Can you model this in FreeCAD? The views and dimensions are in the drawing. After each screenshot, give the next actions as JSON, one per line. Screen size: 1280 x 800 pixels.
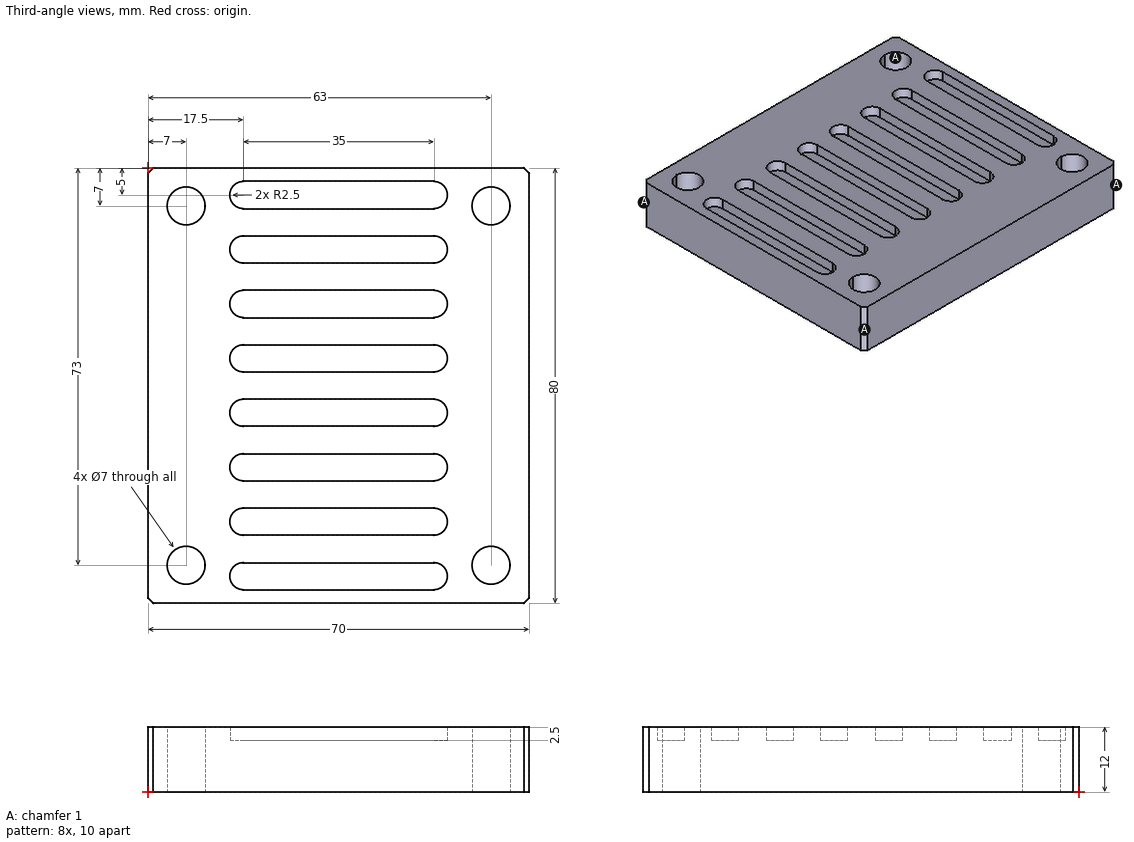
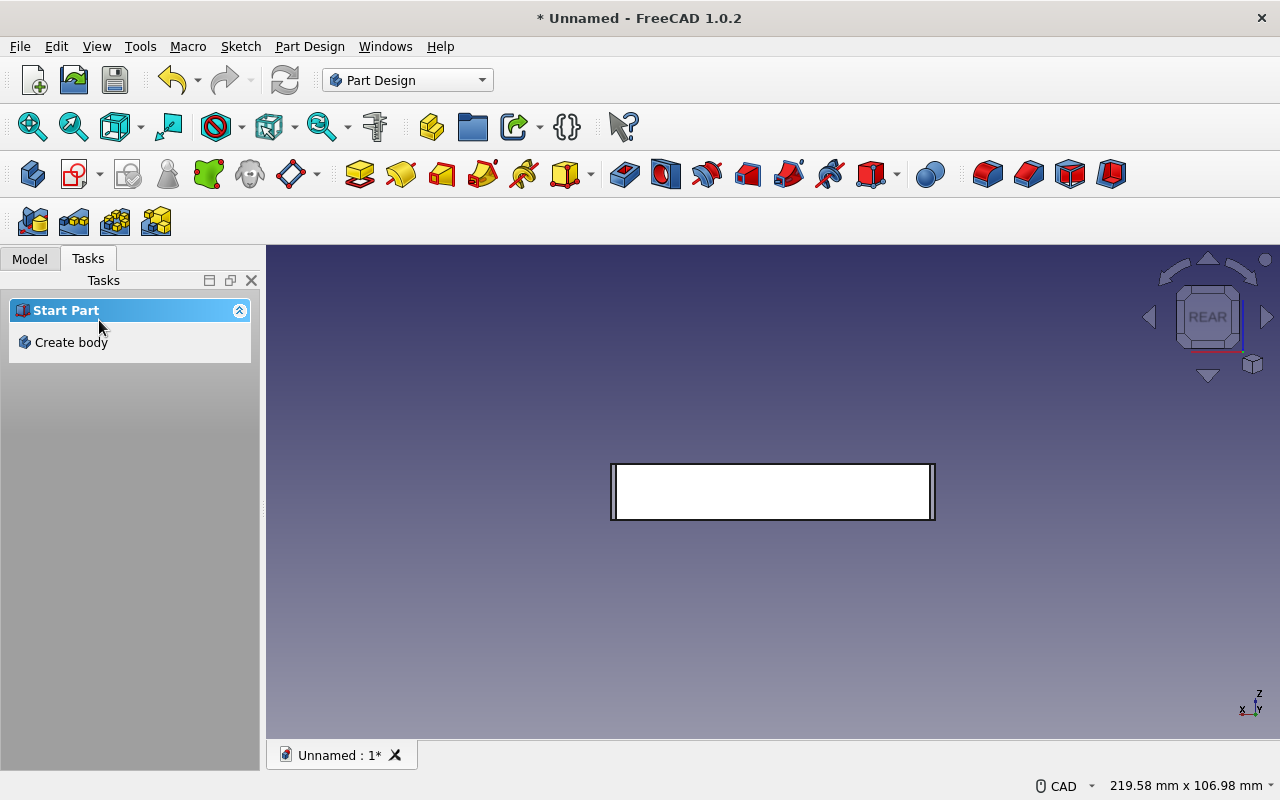
{"action": "key", "text": "0"}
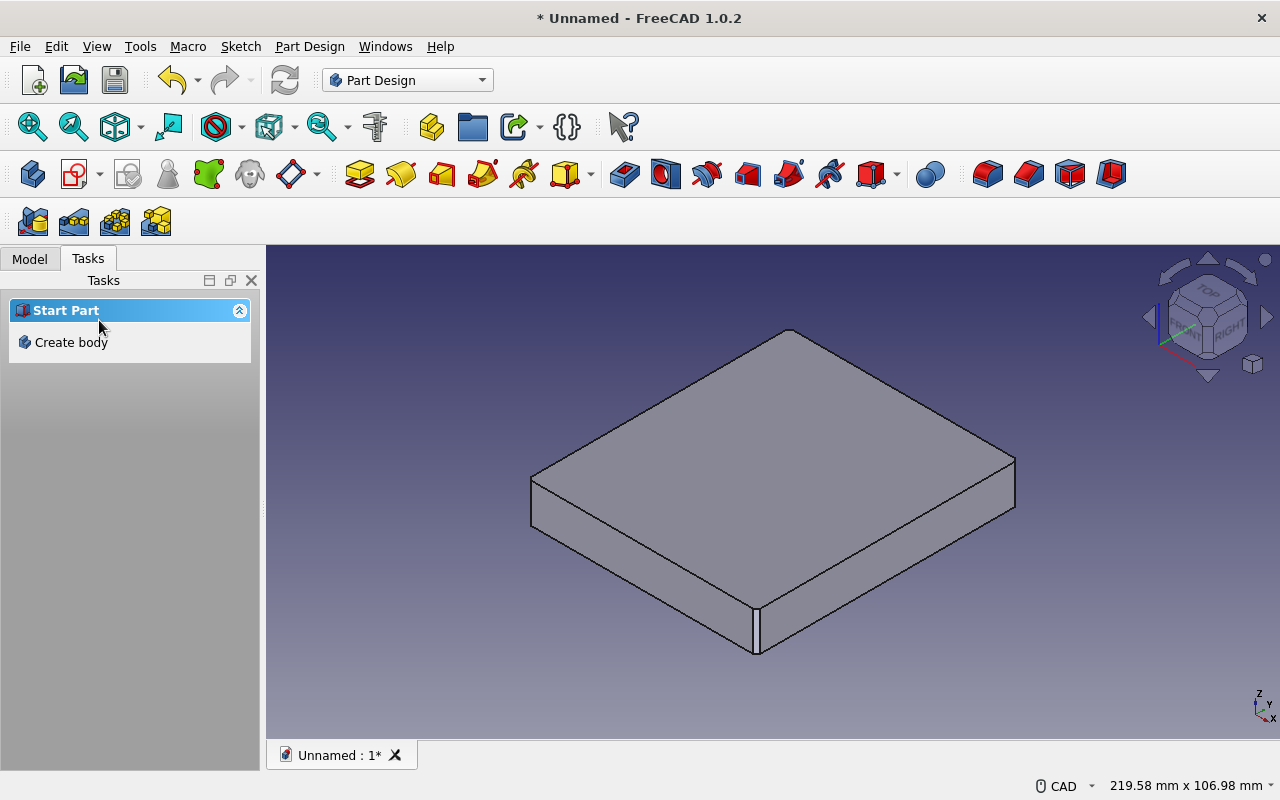
{"action": "left_click", "coordinate": [773, 468]}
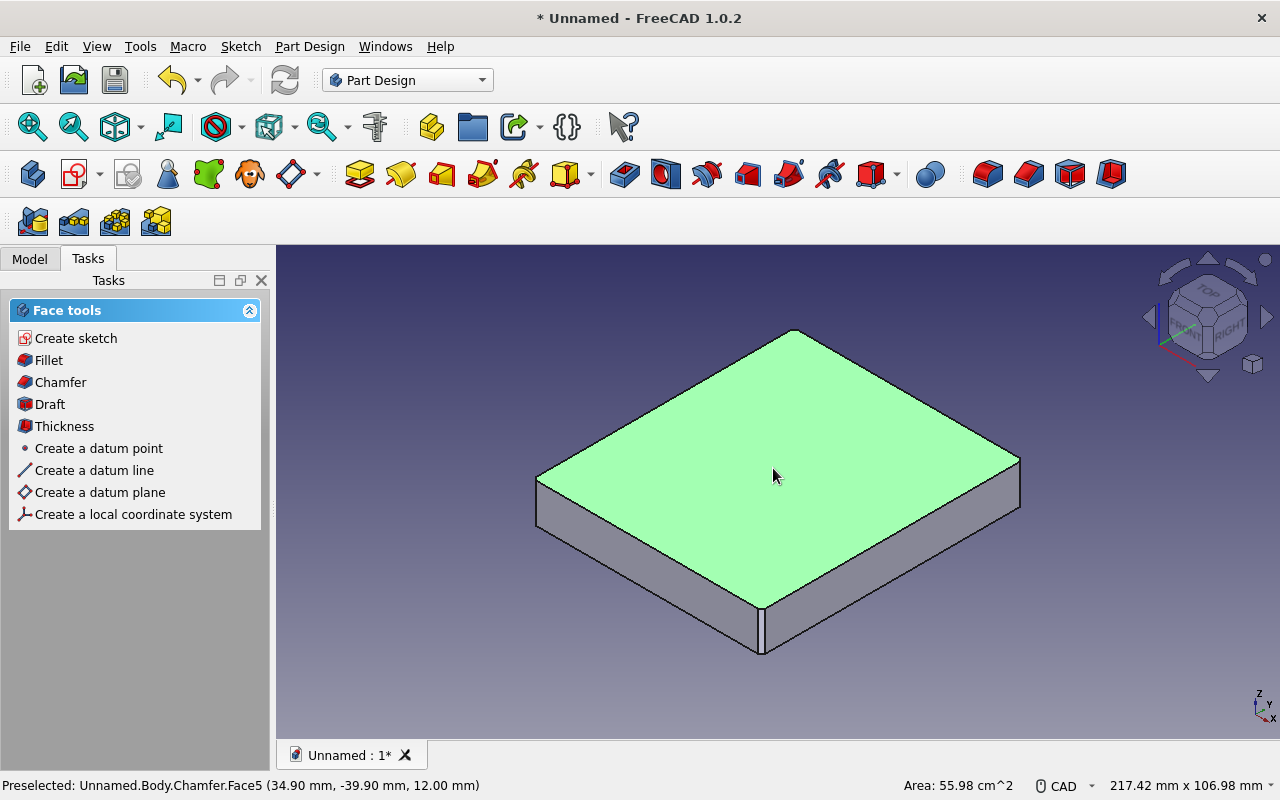
{"action": "left_click", "coordinate": [74, 174]}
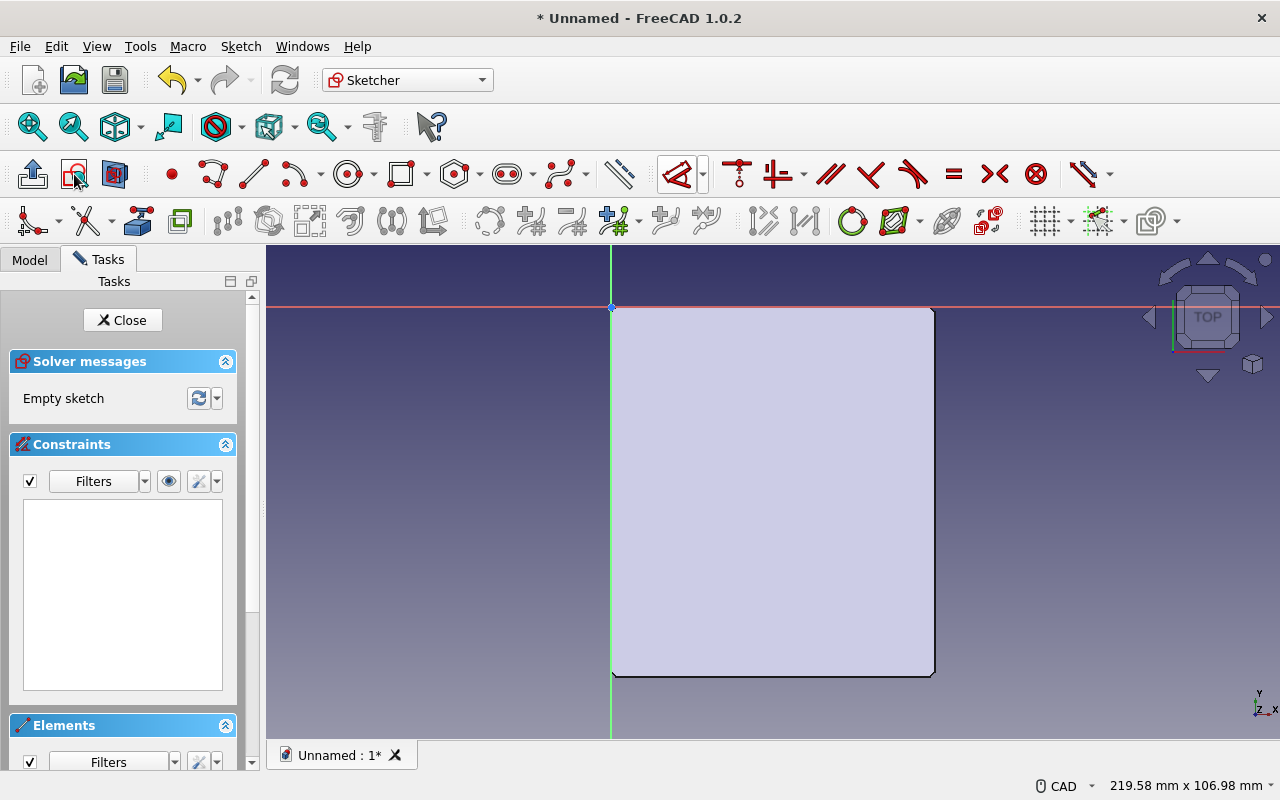
{"action": "scroll", "coordinate": [766, 273], "scroll_direction": "up", "scroll_amount": 4}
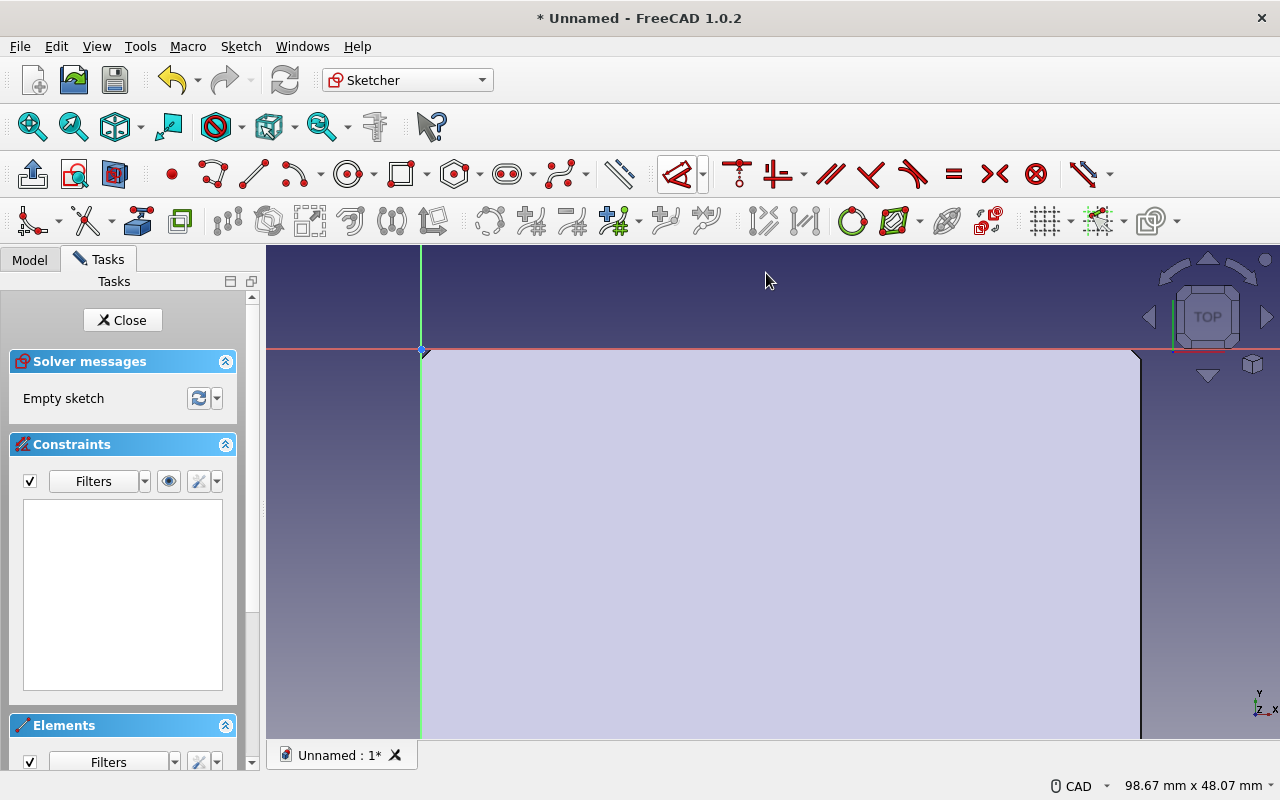
{"action": "key", "text": "g s"}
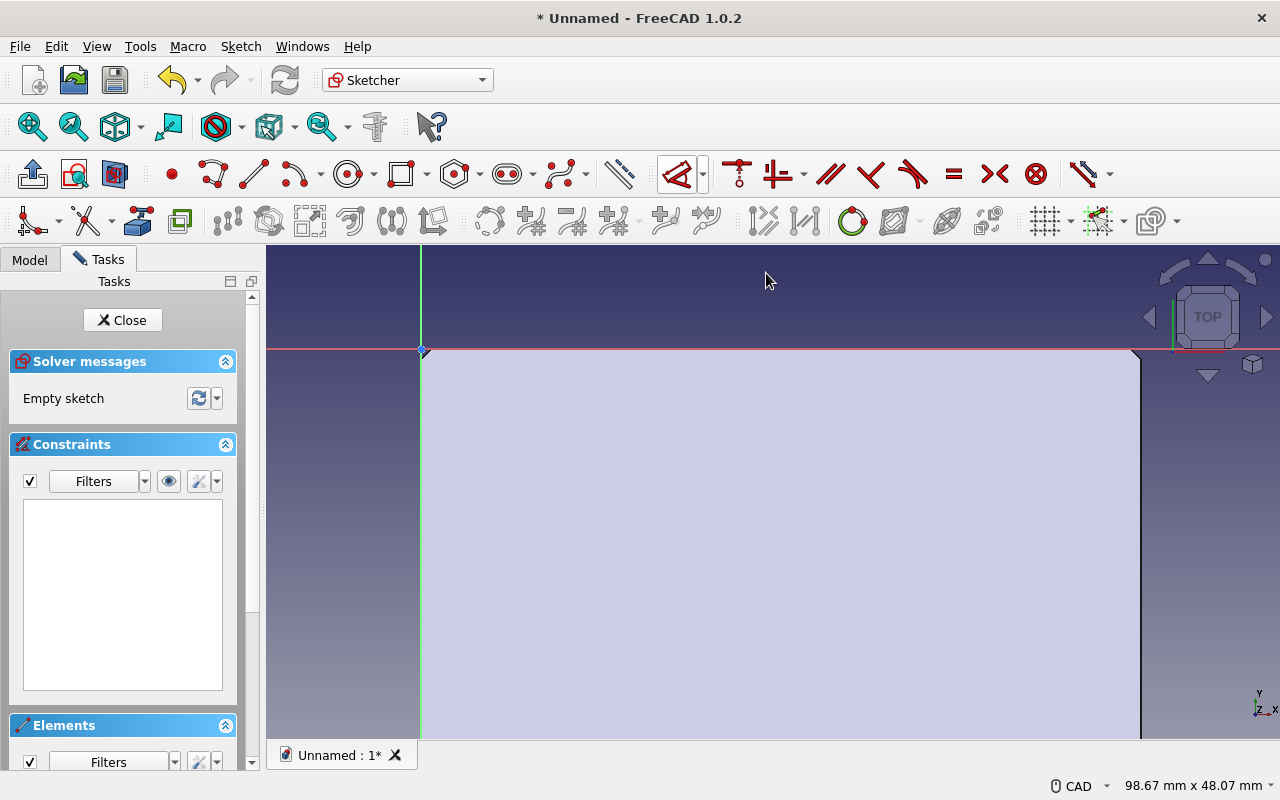
{"action": "left_click", "coordinate": [601, 401]}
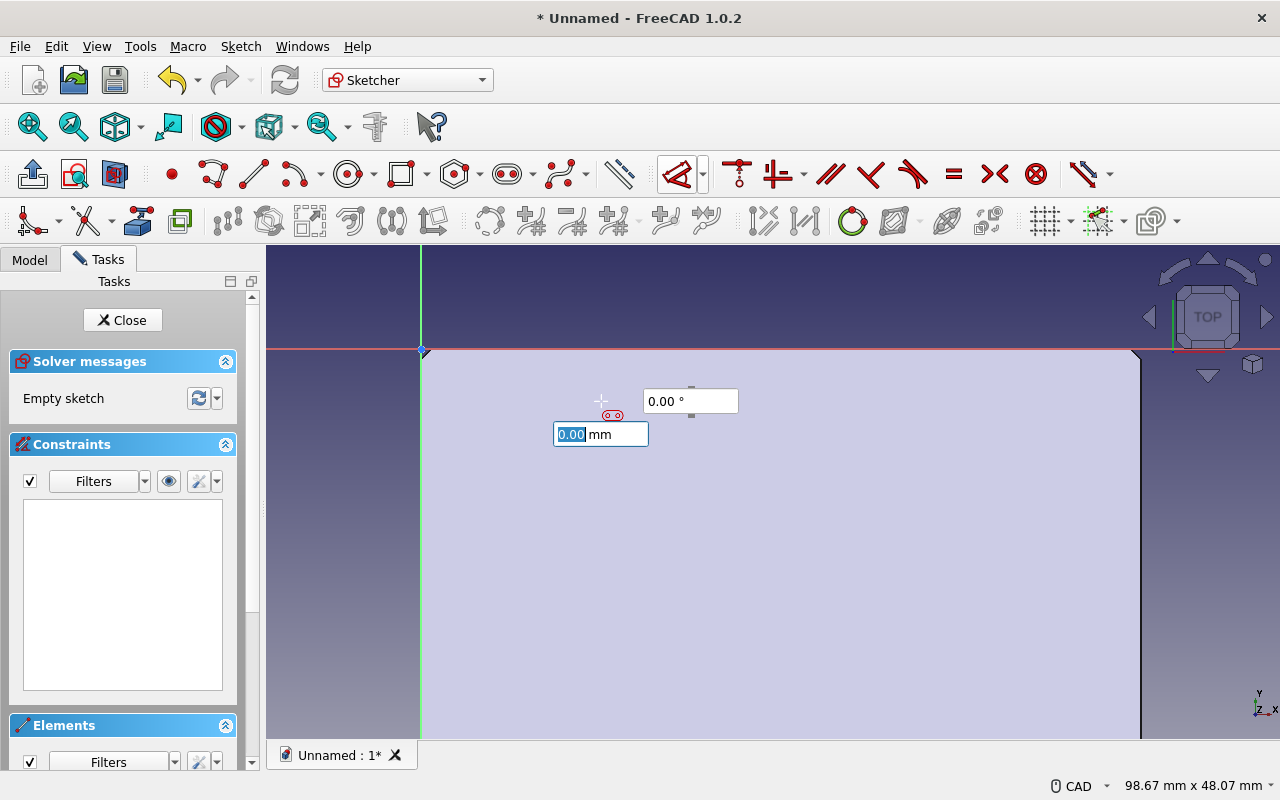
{"action": "left_click", "coordinate": [961, 401]}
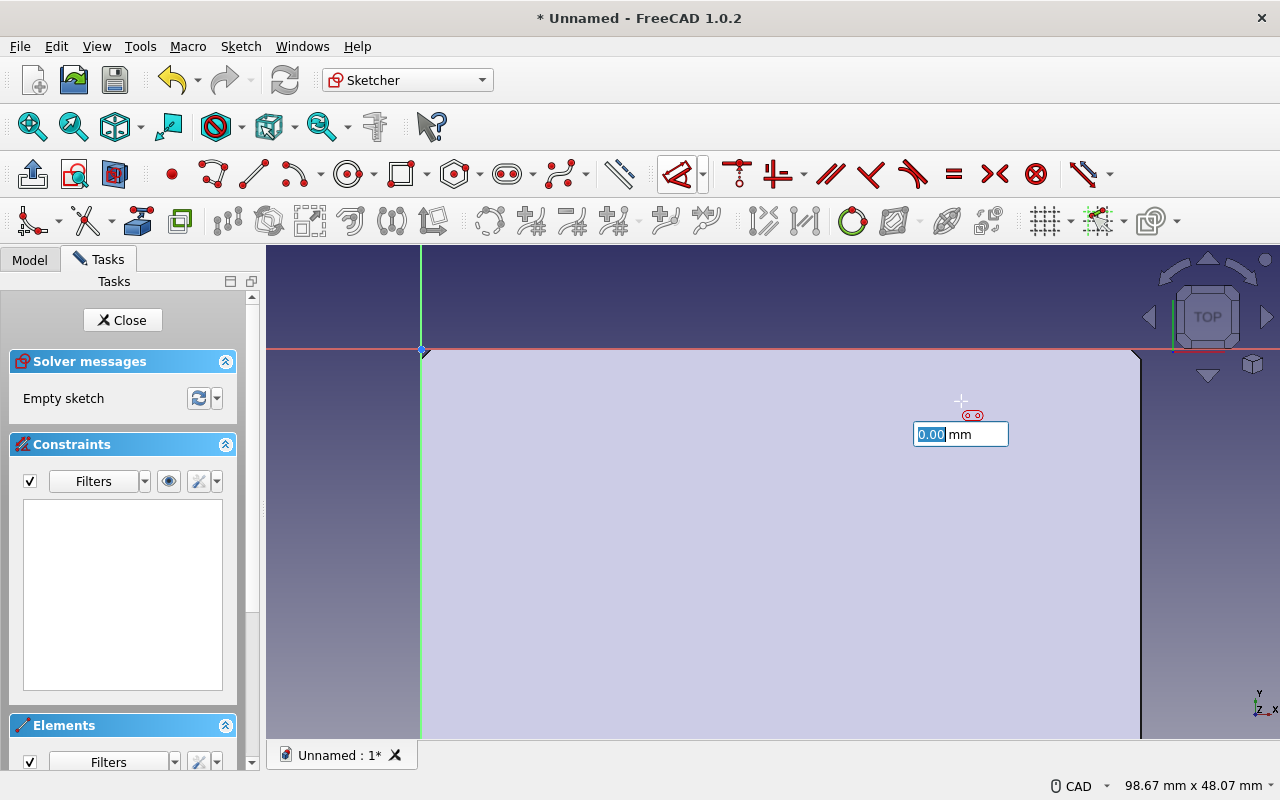
{"action": "left_click", "coordinate": [781, 375]}
{"action": "key", "text": "Escape"}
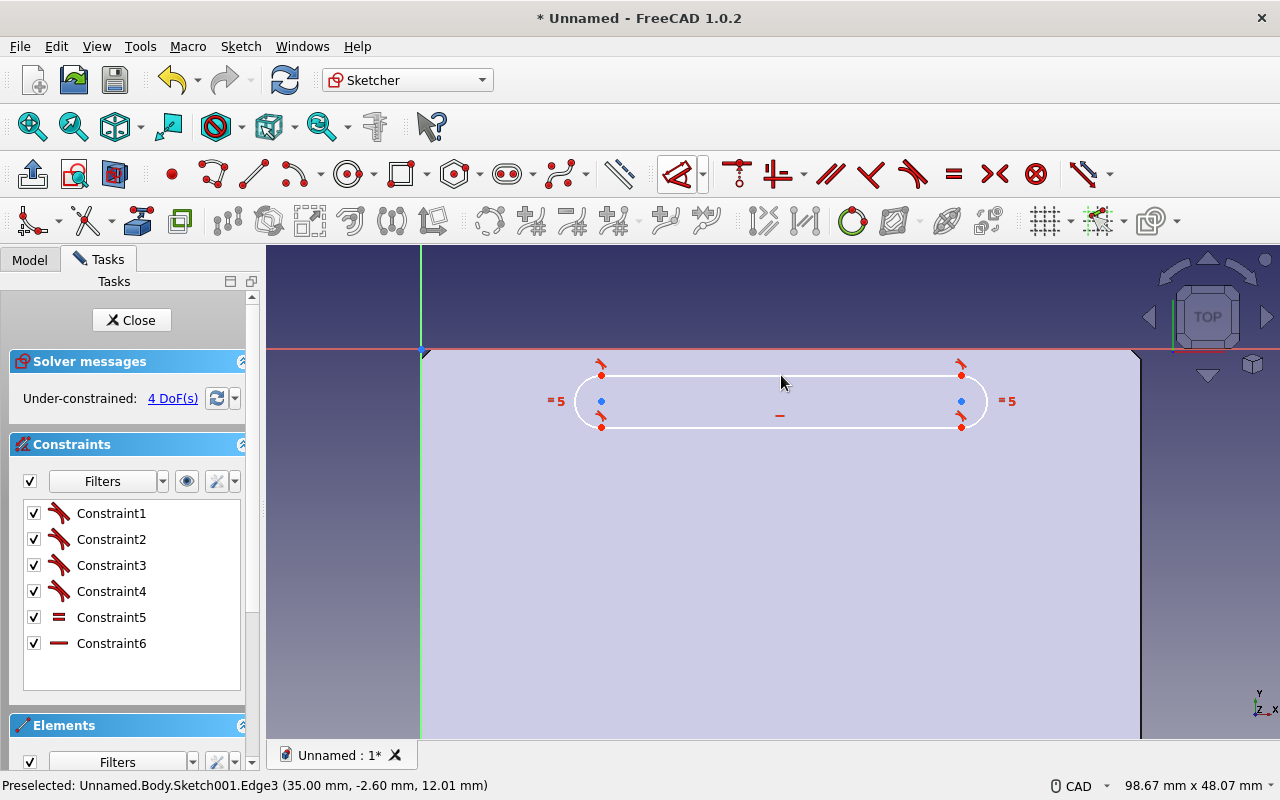
{"action": "key", "text": "d"}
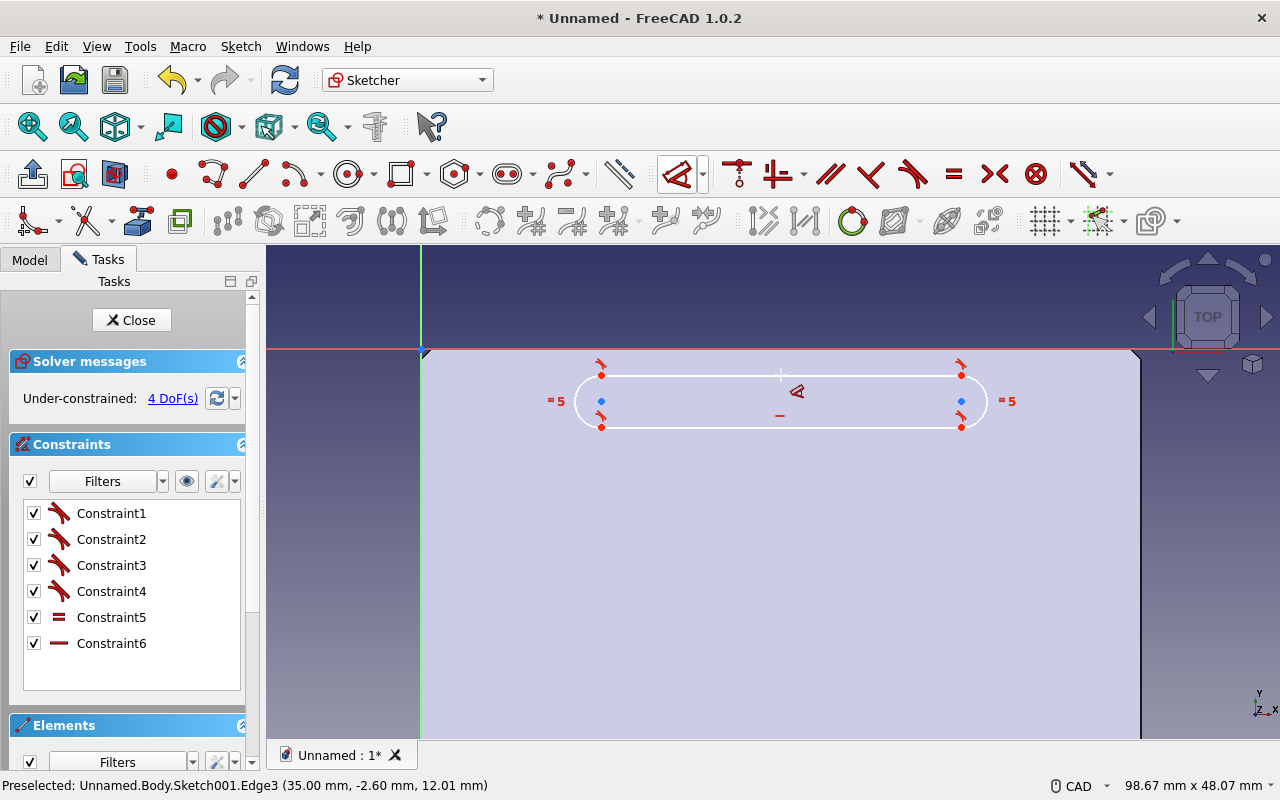
{"action": "scroll", "coordinate": [580, 387], "scroll_direction": "up", "scroll_amount": 3}